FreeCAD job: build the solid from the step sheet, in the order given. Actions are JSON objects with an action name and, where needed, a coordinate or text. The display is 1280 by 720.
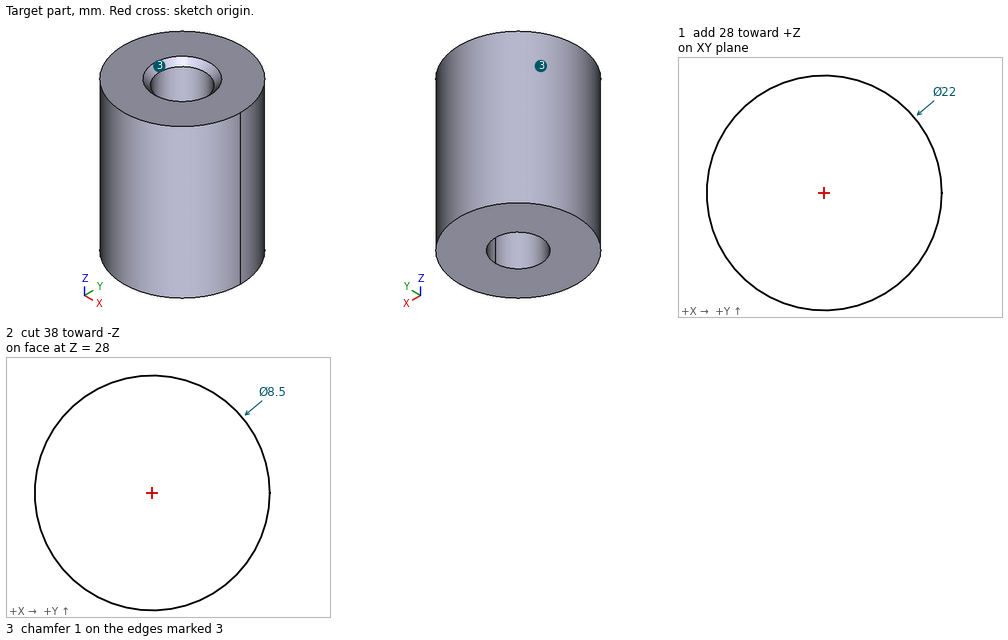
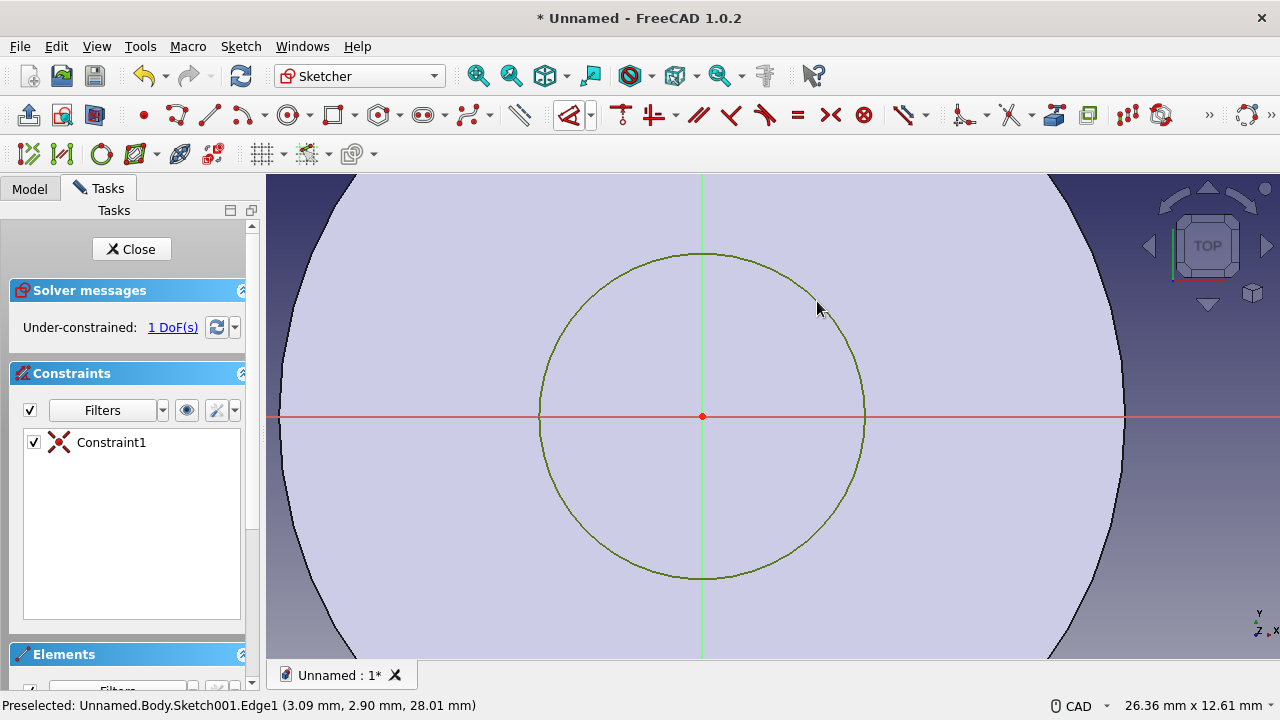
{"action": "key", "text": "k o"}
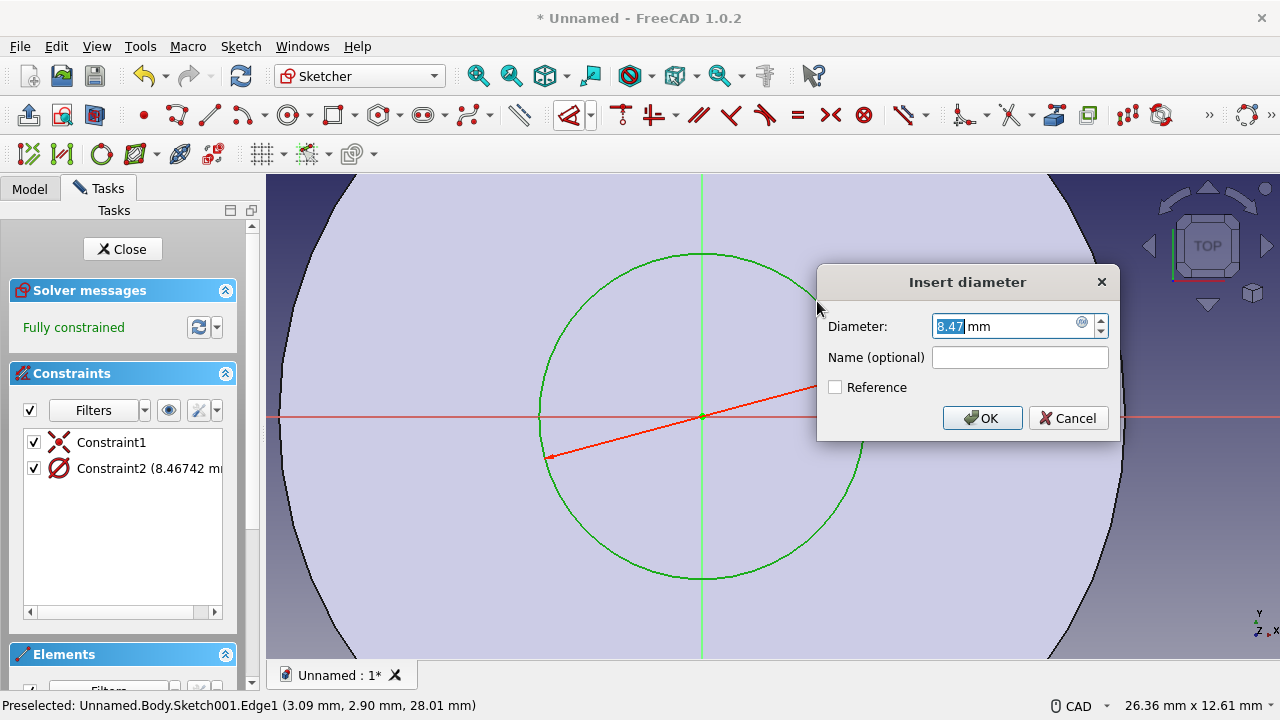
{"action": "type", "text": "8.5"}
{"action": "key", "text": "Return"}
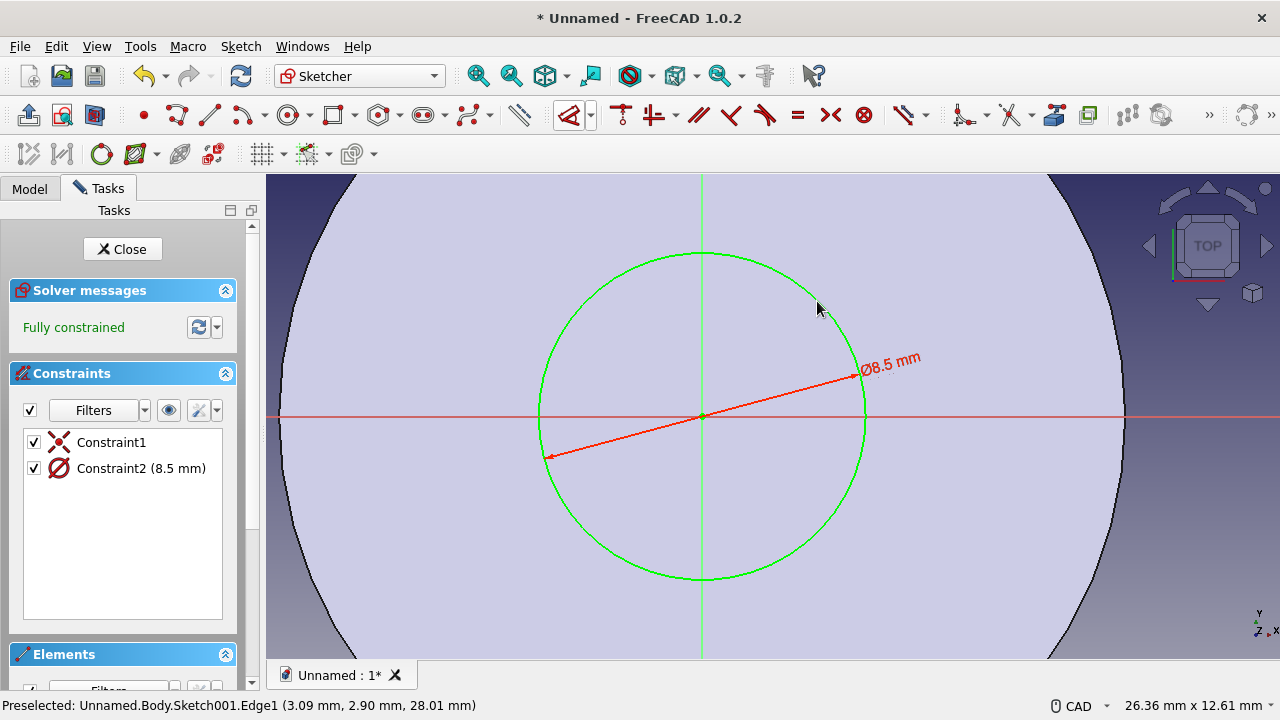
{"action": "left_click", "coordinate": [123, 249]}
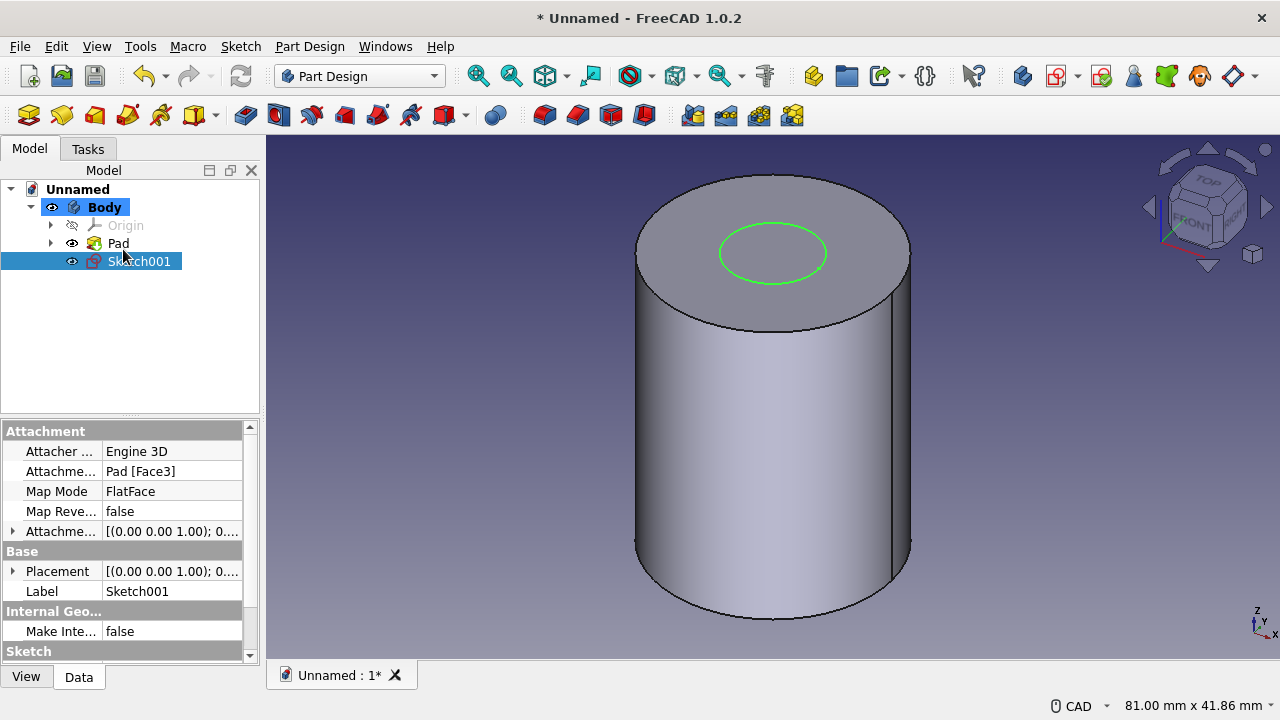
{"action": "left_click", "coordinate": [246, 116]}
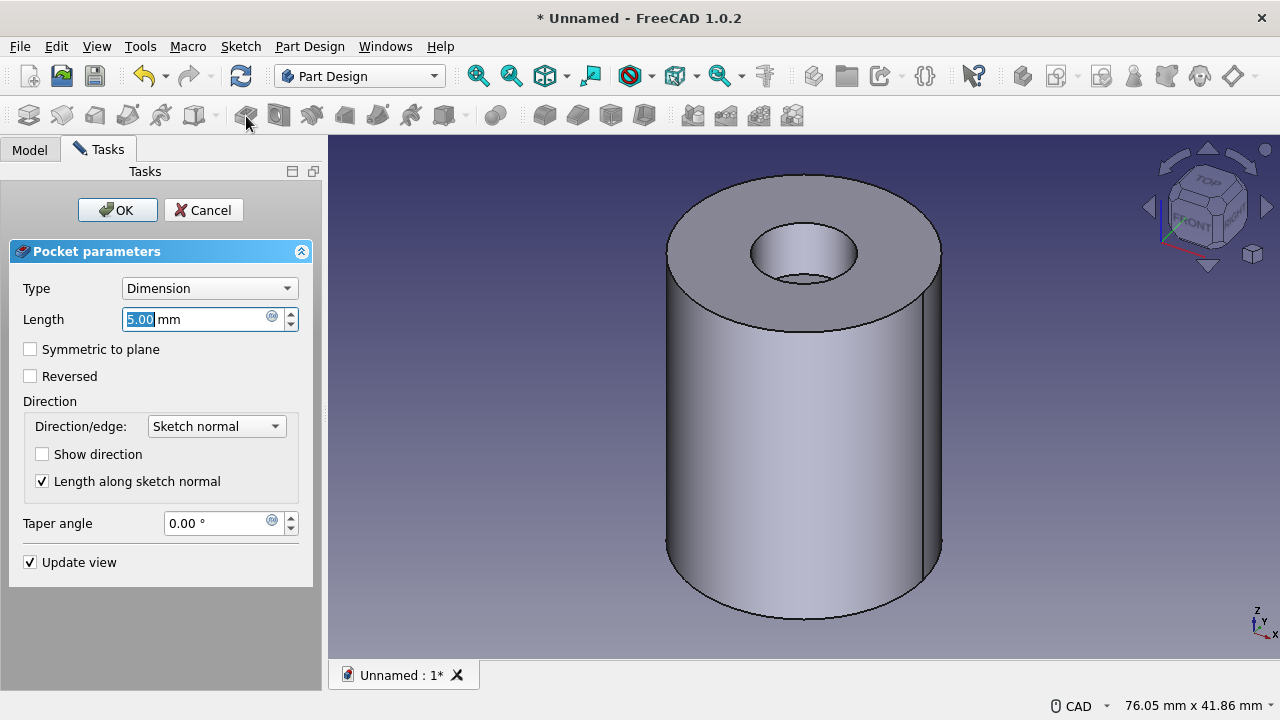
{"action": "type", "text": "38"}
{"action": "key", "text": "Tab"}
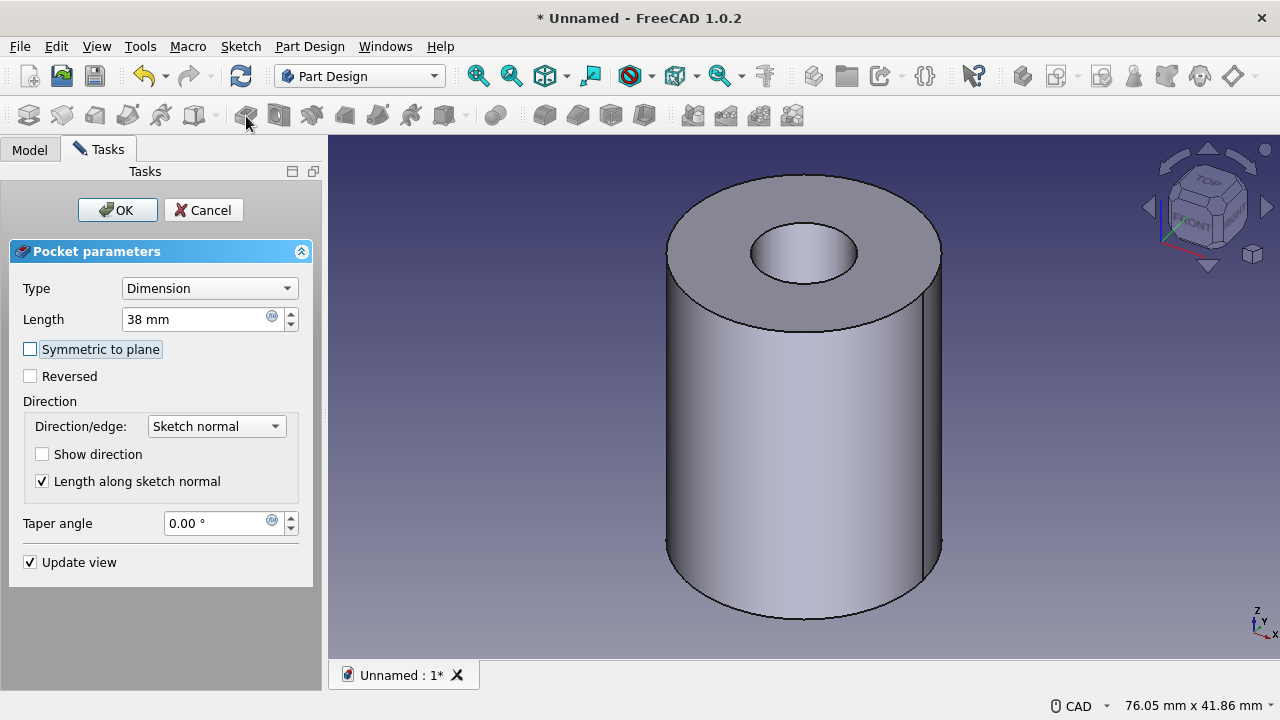
{"action": "left_click", "coordinate": [118, 210]}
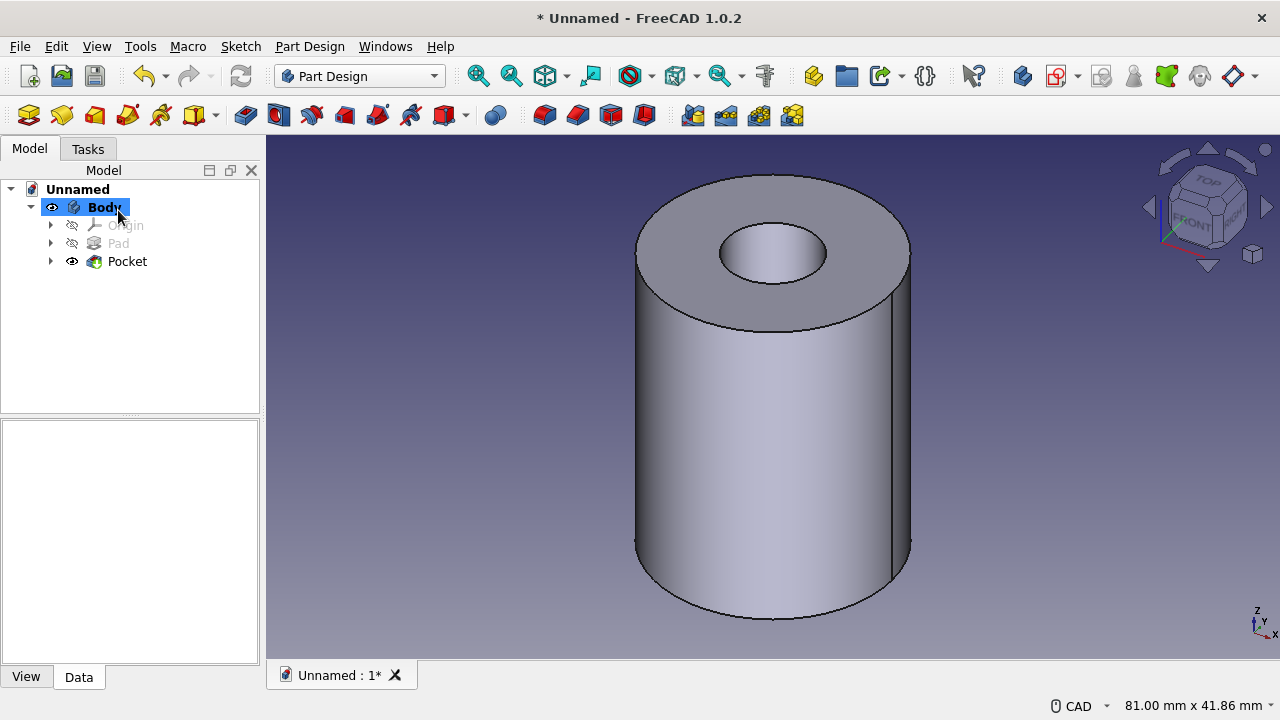
{"action": "left_click", "coordinate": [727, 237]}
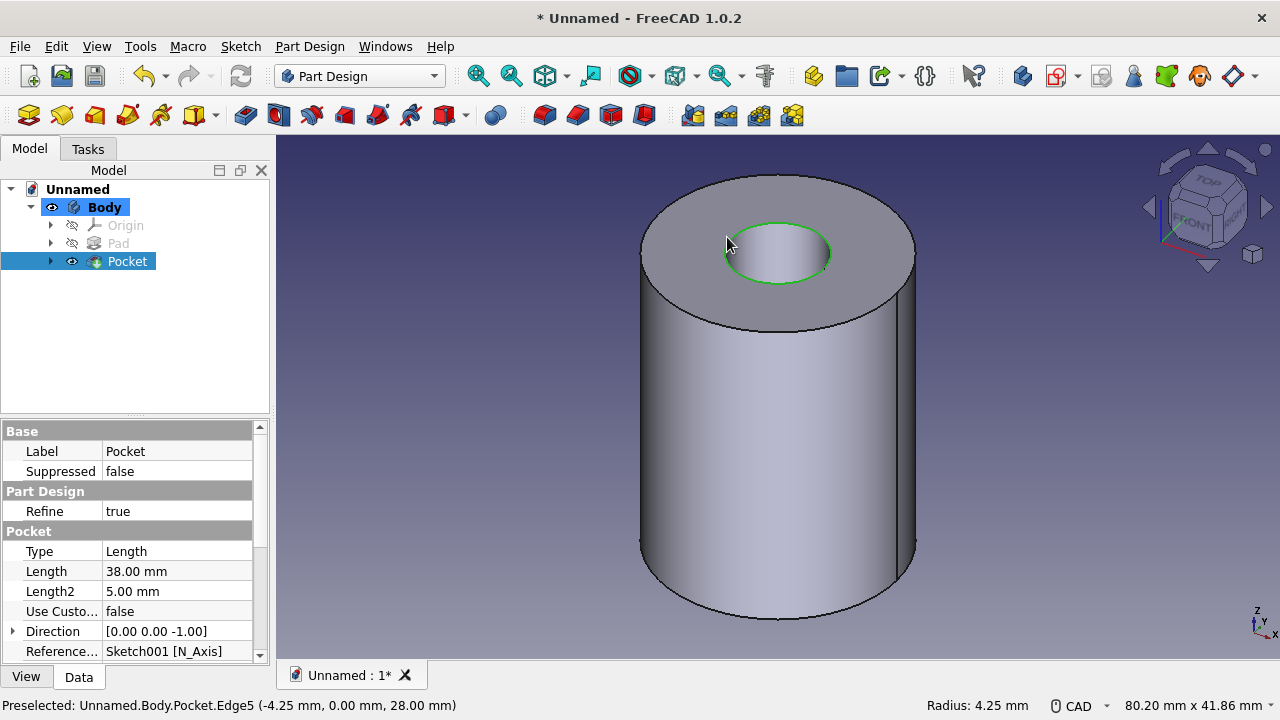
{"action": "left_click", "coordinate": [578, 116]}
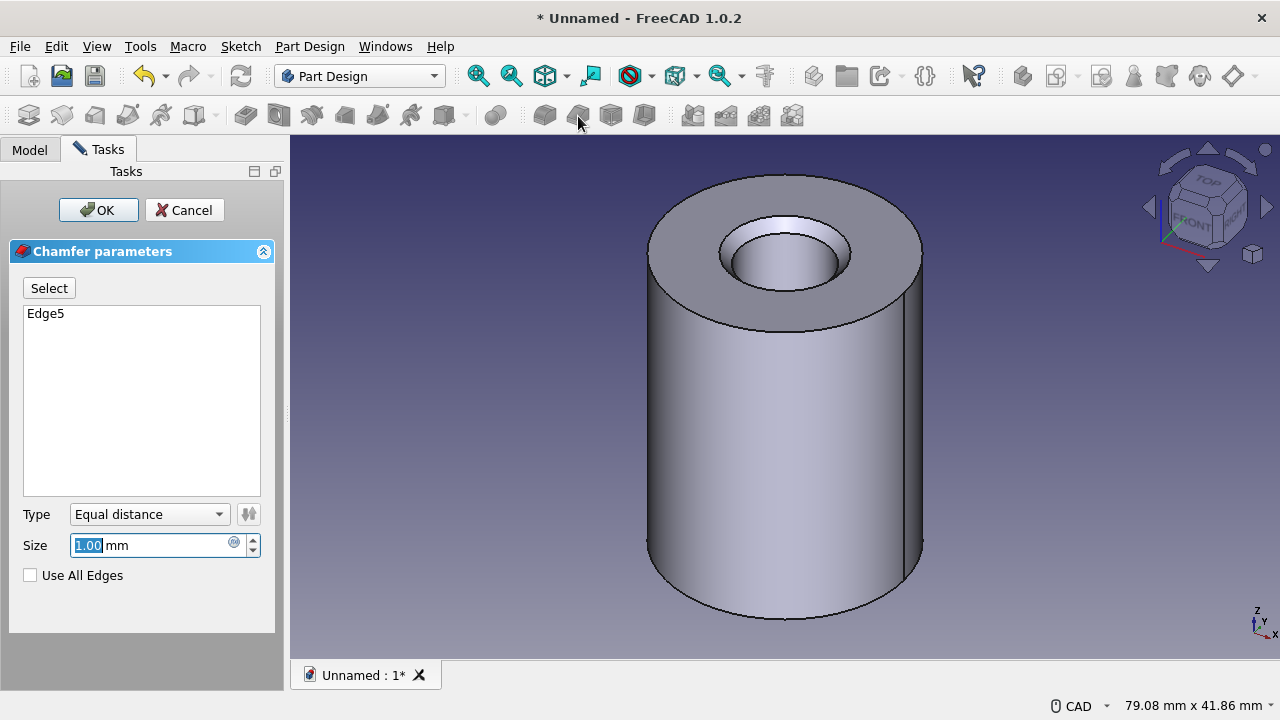
{"action": "type", "text": "1"}
{"action": "key", "text": "Tab"}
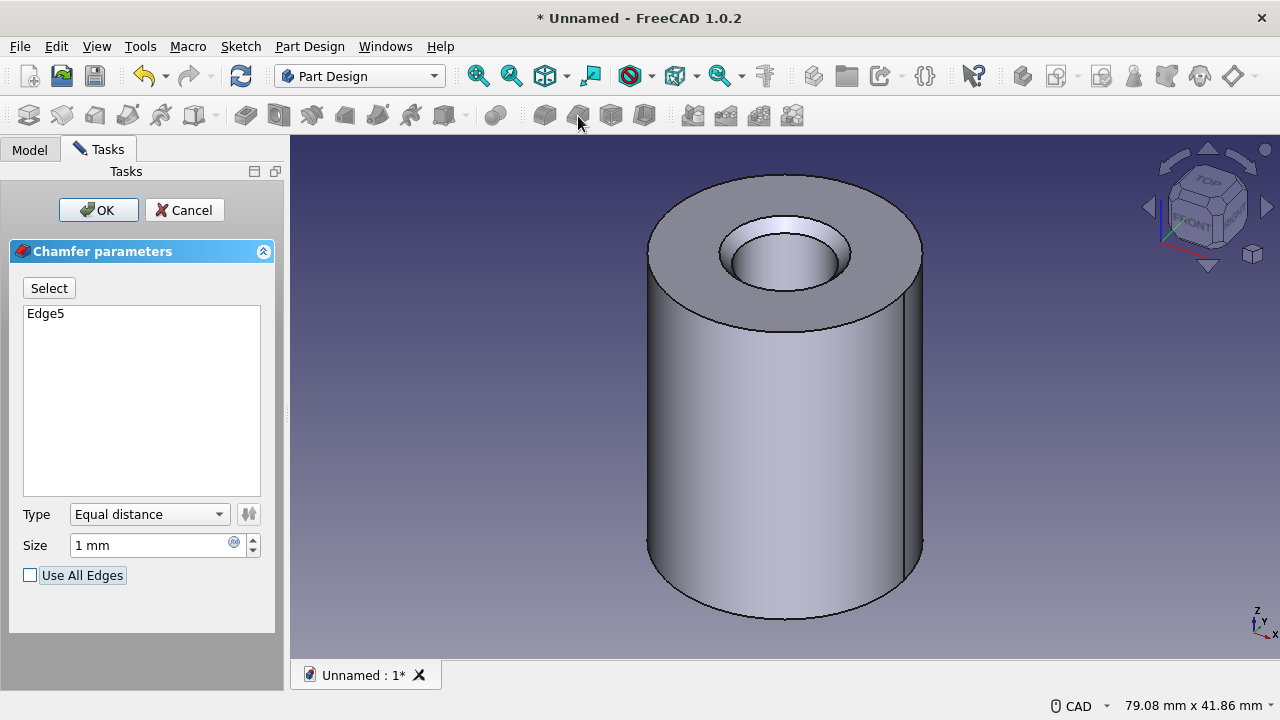
{"action": "left_click", "coordinate": [99, 210]}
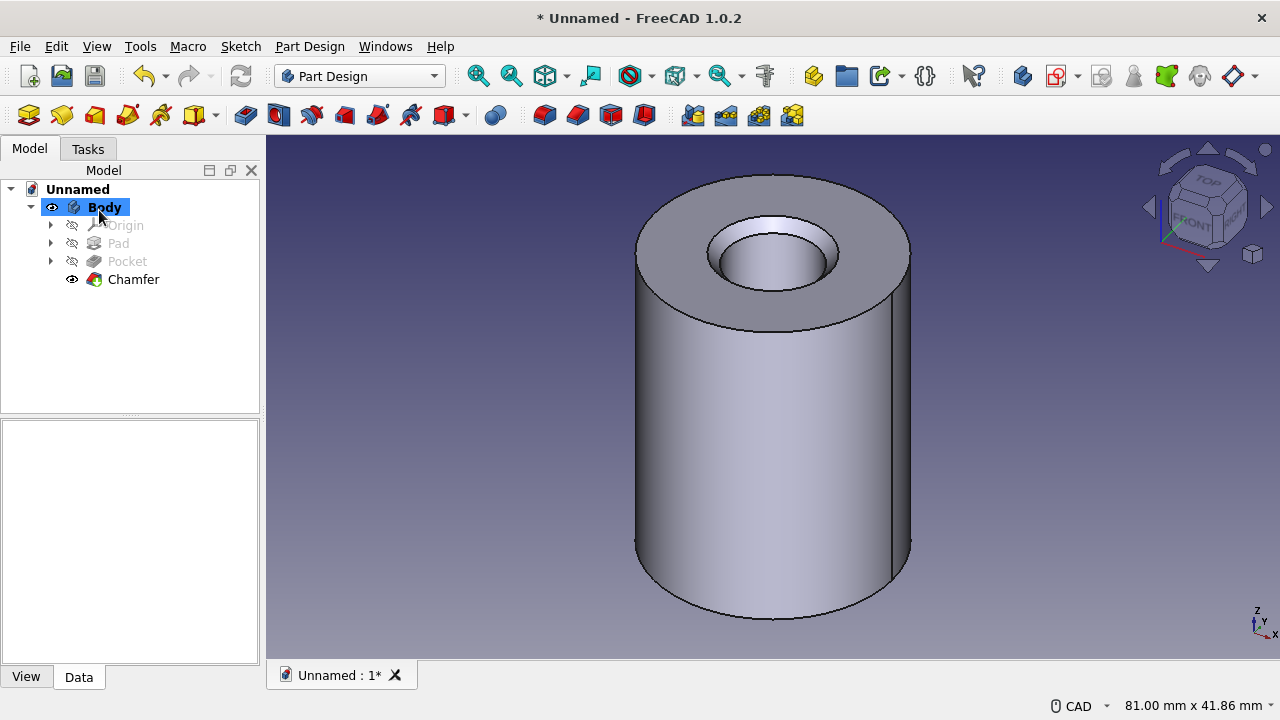
{"action": "key", "text": "0"}